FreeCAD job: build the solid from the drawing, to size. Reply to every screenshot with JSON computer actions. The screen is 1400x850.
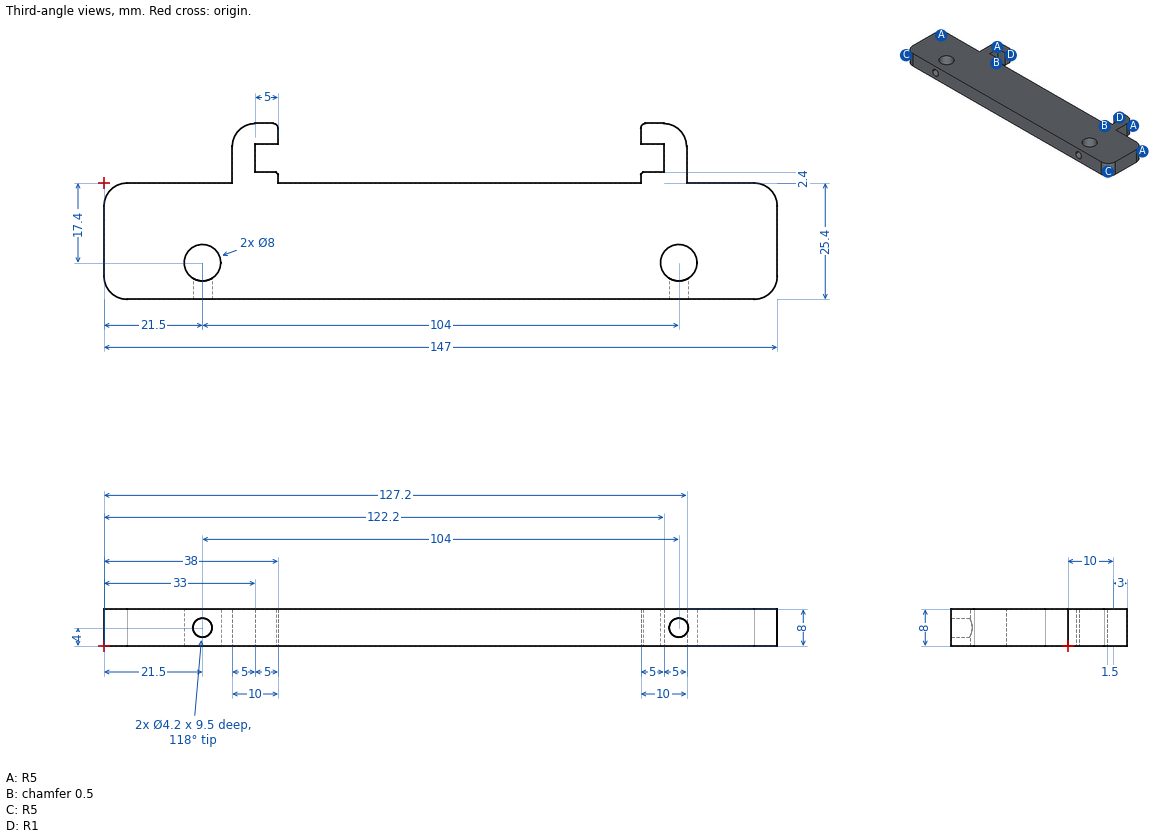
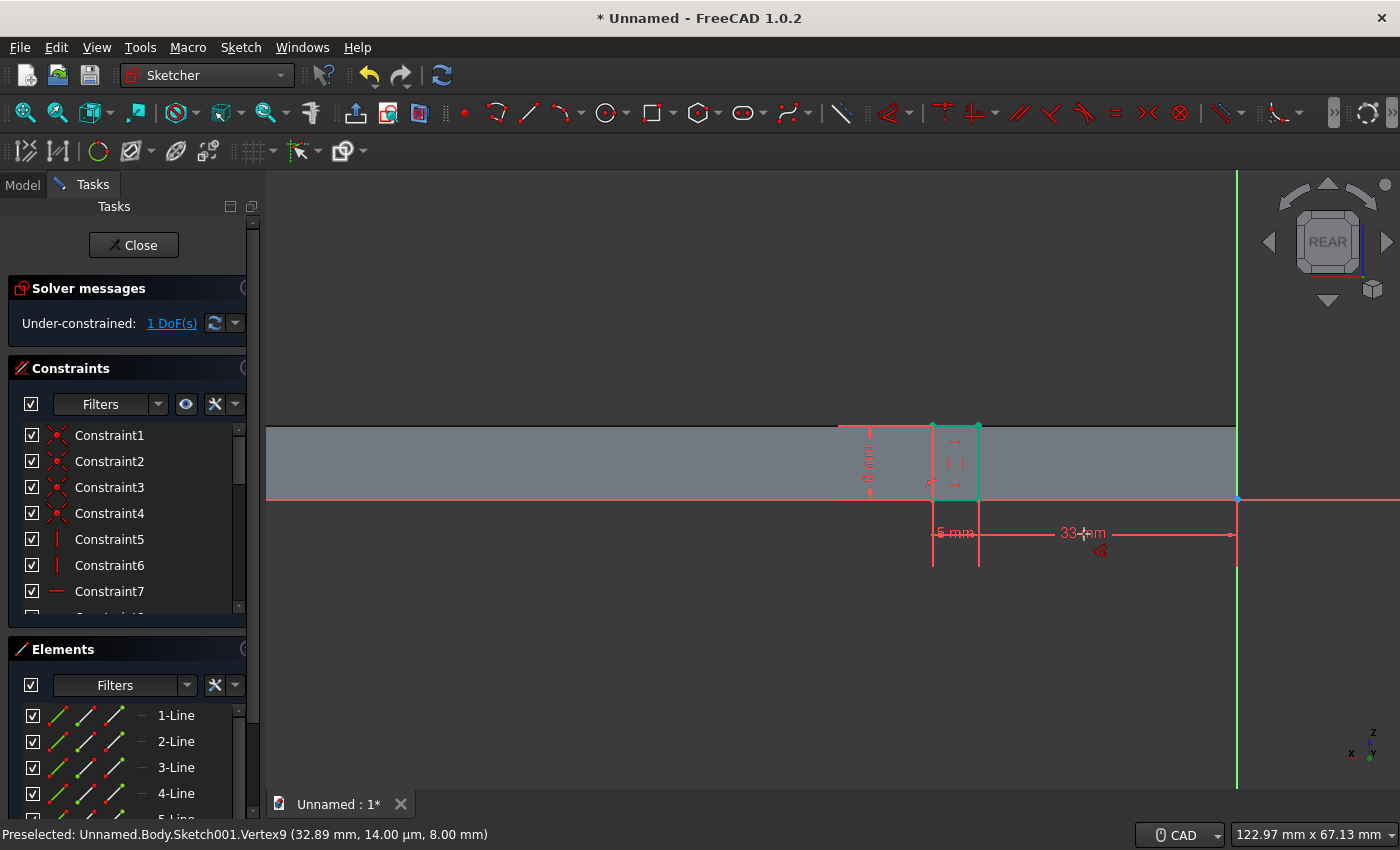
{"action": "scroll", "coordinate": [903, 500], "scroll_direction": "down", "scroll_amount": 3}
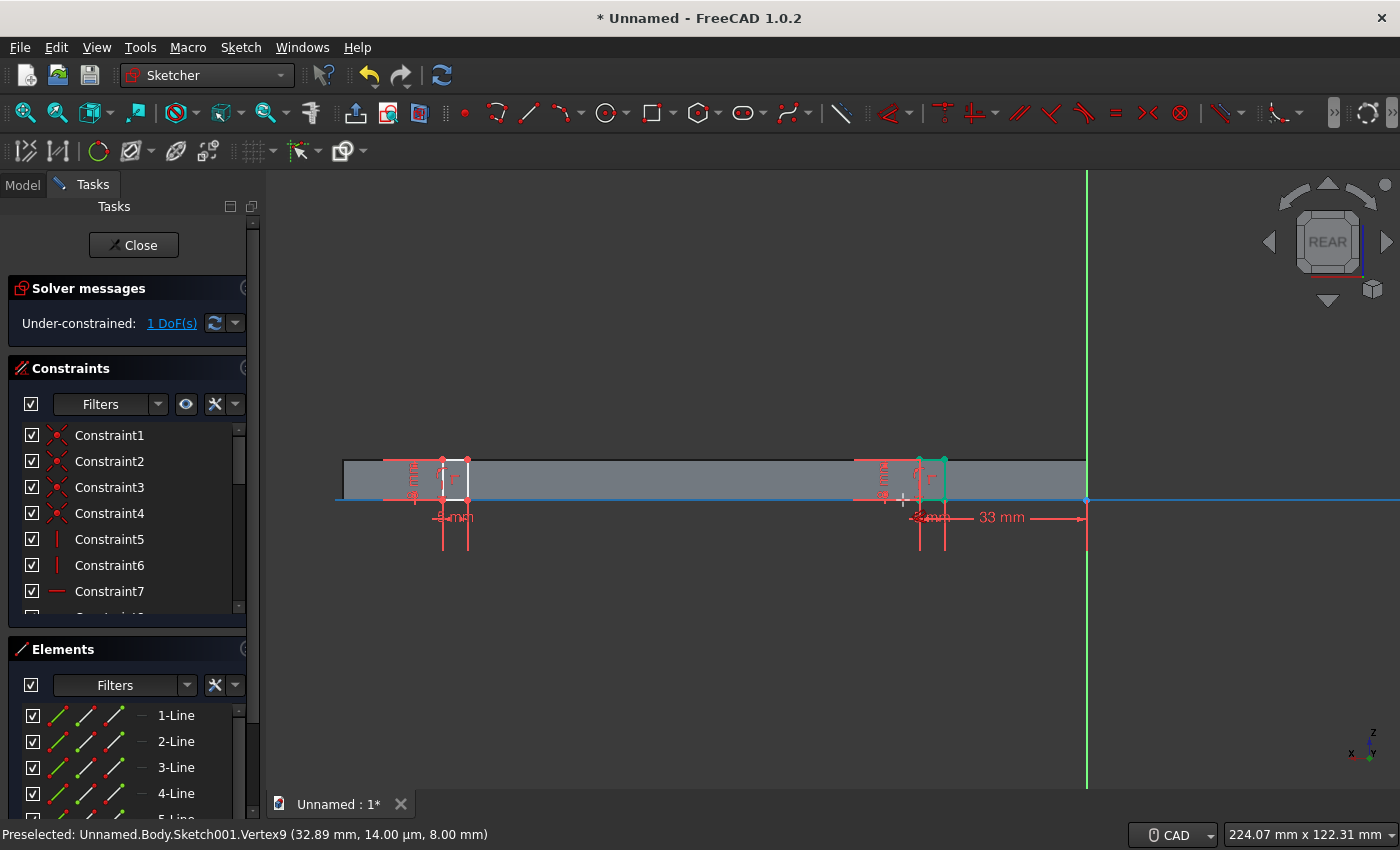
{"action": "left_click", "coordinate": [443, 460]}
{"action": "left_click", "coordinate": [765, 534]}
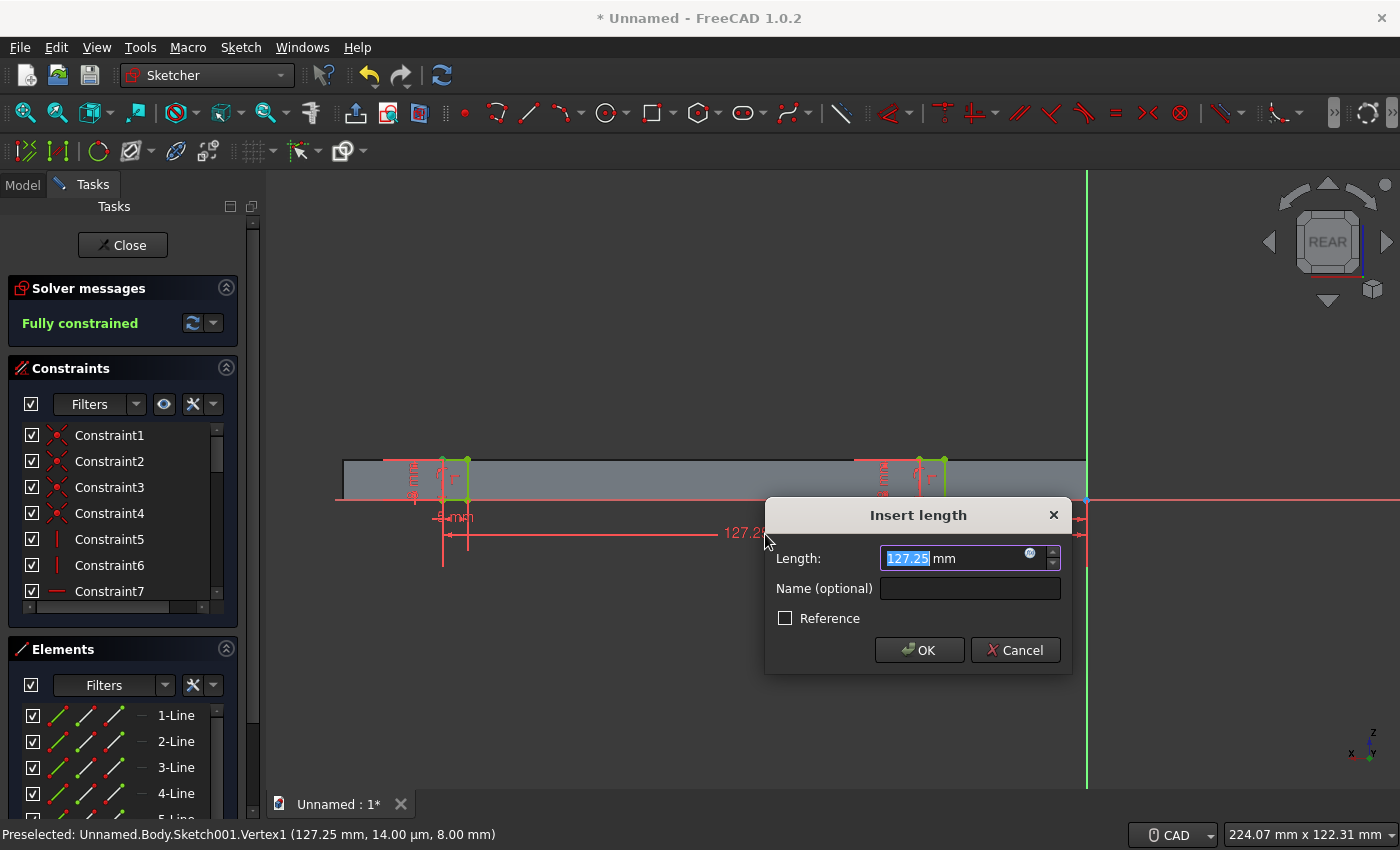
{"action": "type", "text": "127.2"}
{"action": "key", "text": "Return"}
{"action": "key", "text": "Escape"}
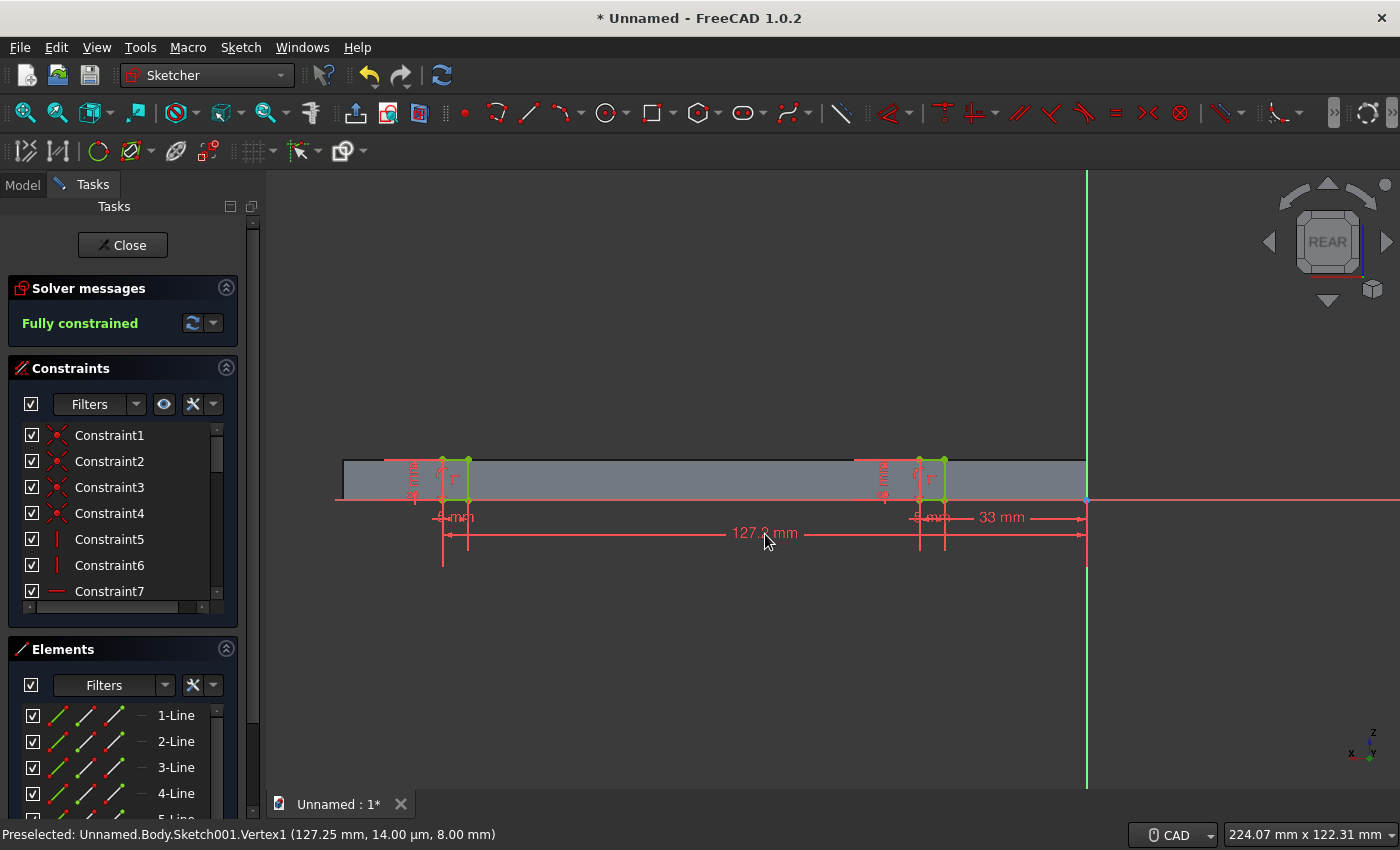
{"action": "left_click", "coordinate": [123, 245]}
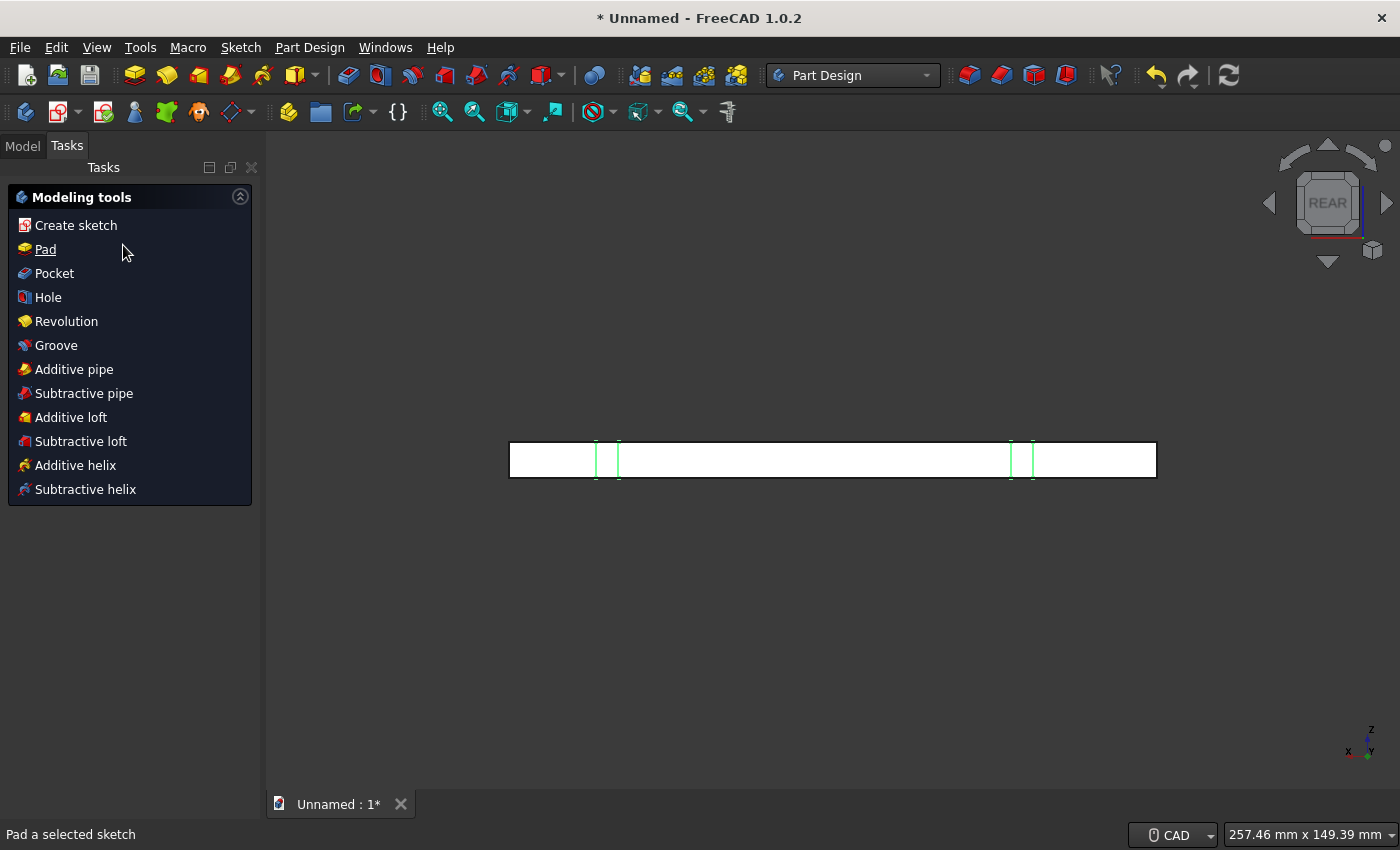
{"action": "left_click", "coordinate": [136, 76]}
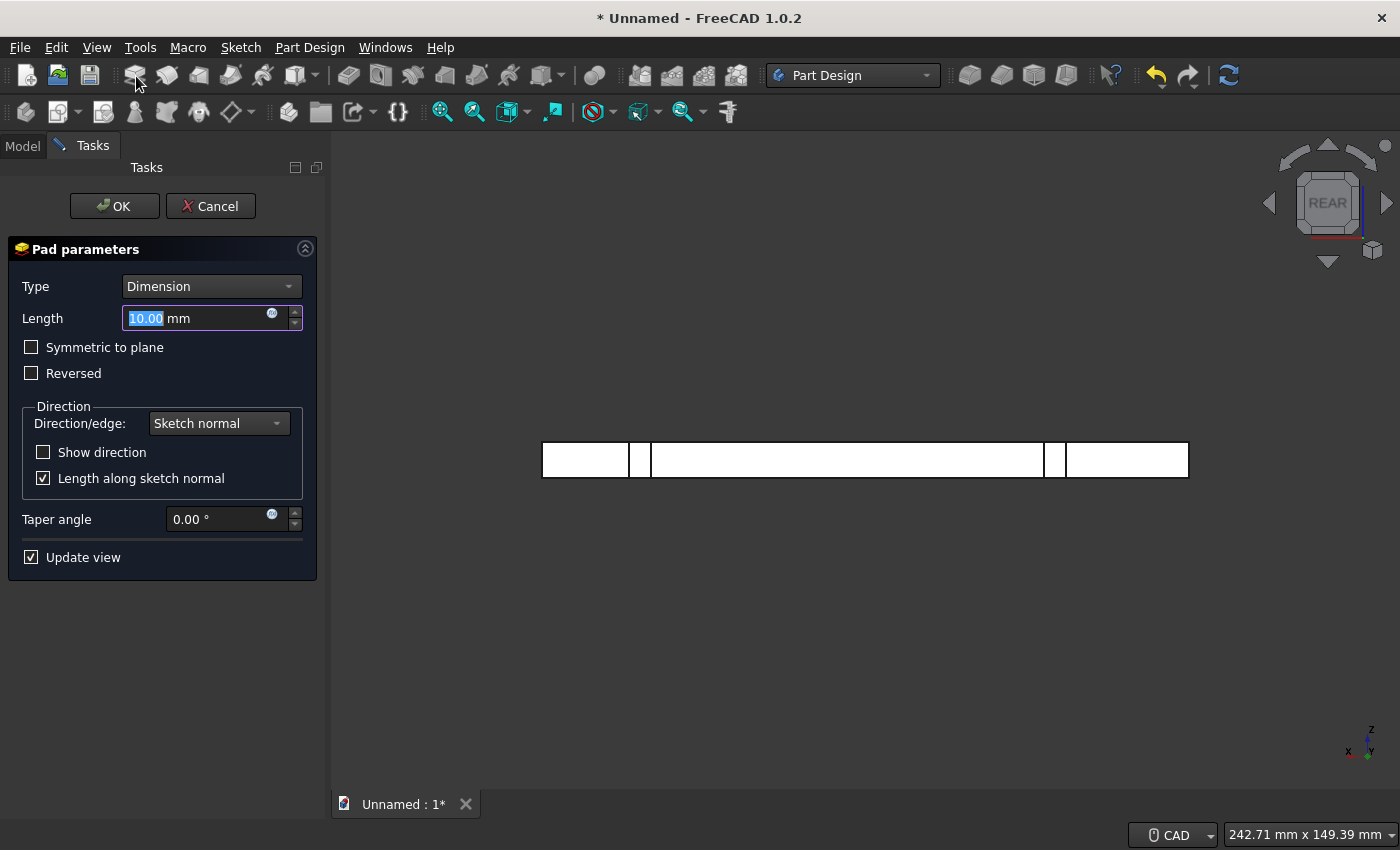
{"action": "type", "text": "10"}
{"action": "key", "text": "Tab"}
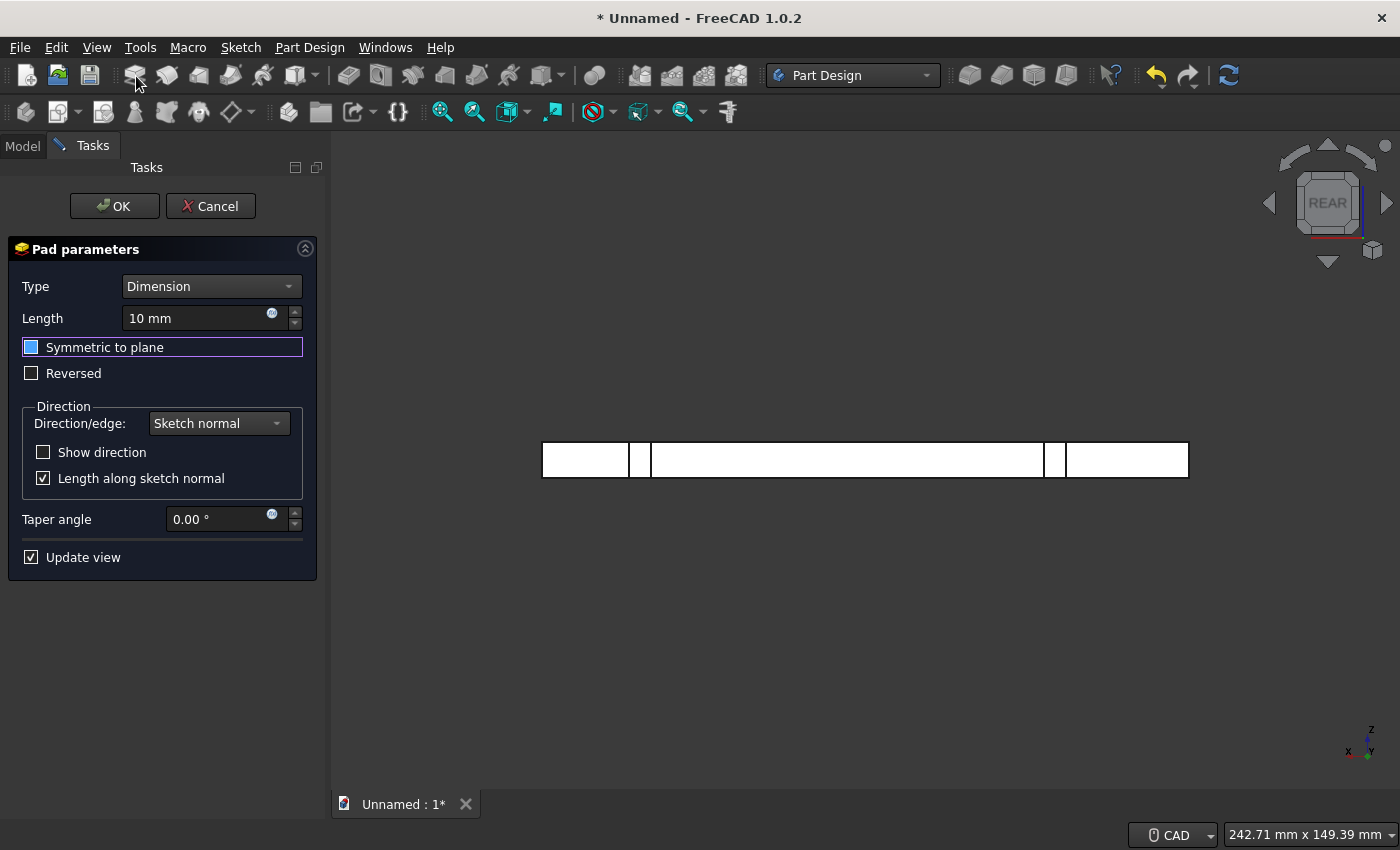
{"action": "left_click", "coordinate": [115, 206]}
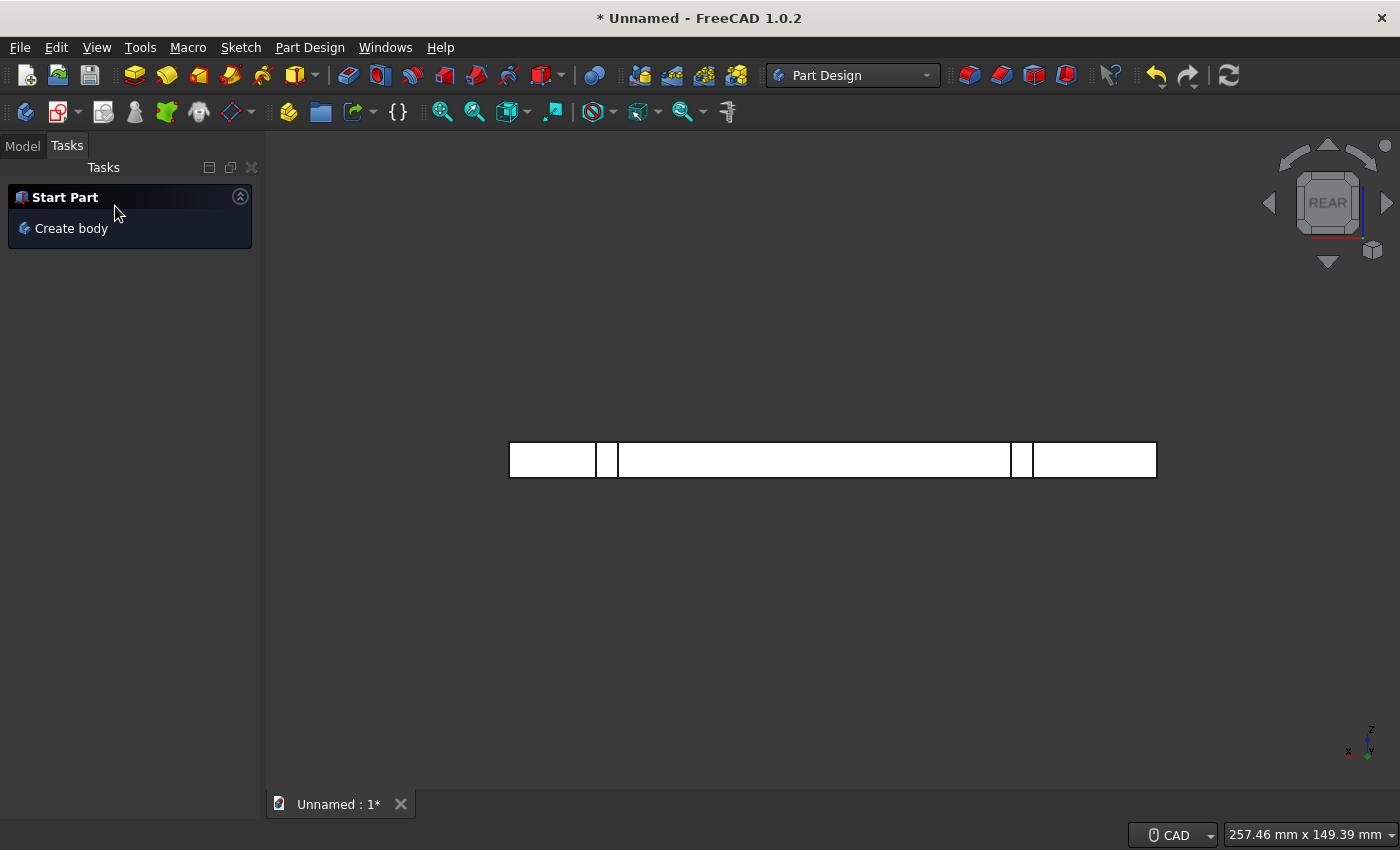
{"action": "left_click", "coordinate": [23, 145]}